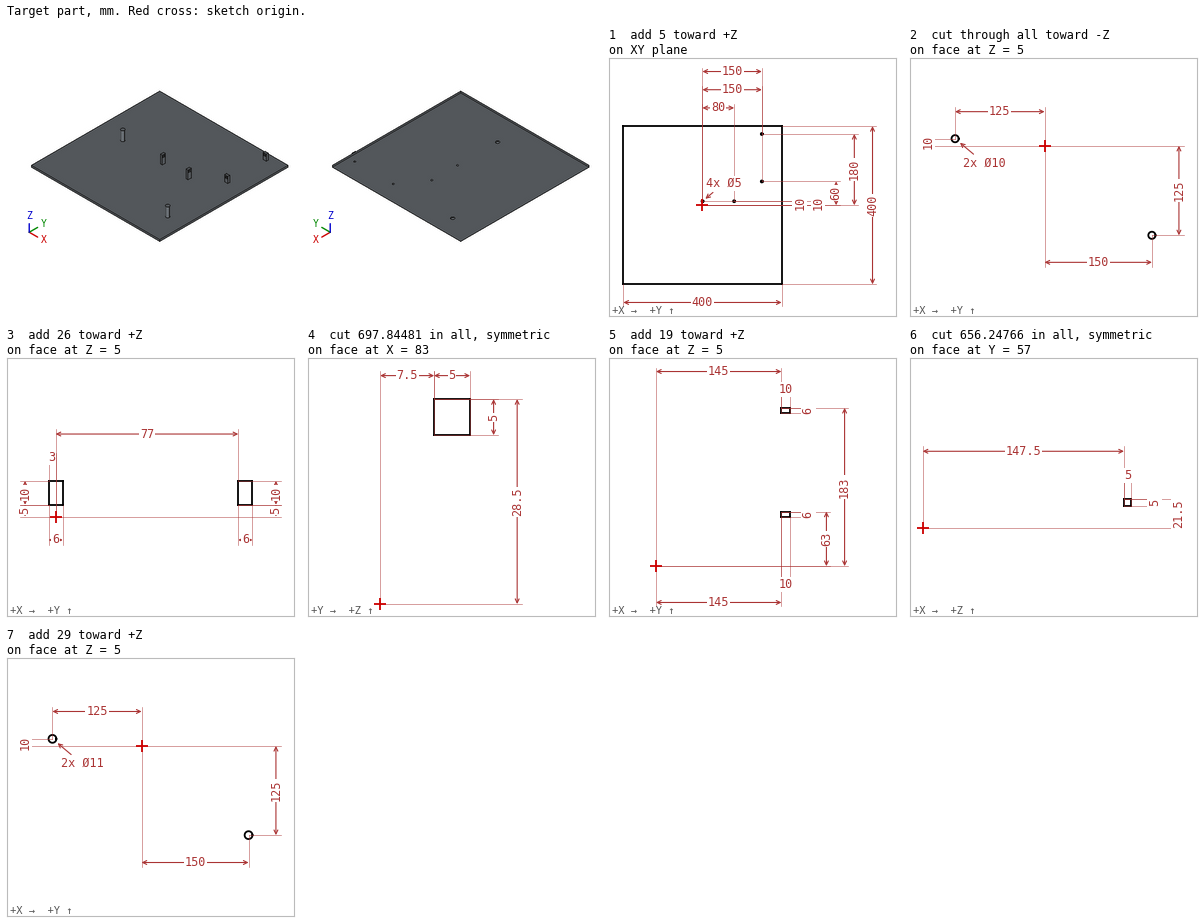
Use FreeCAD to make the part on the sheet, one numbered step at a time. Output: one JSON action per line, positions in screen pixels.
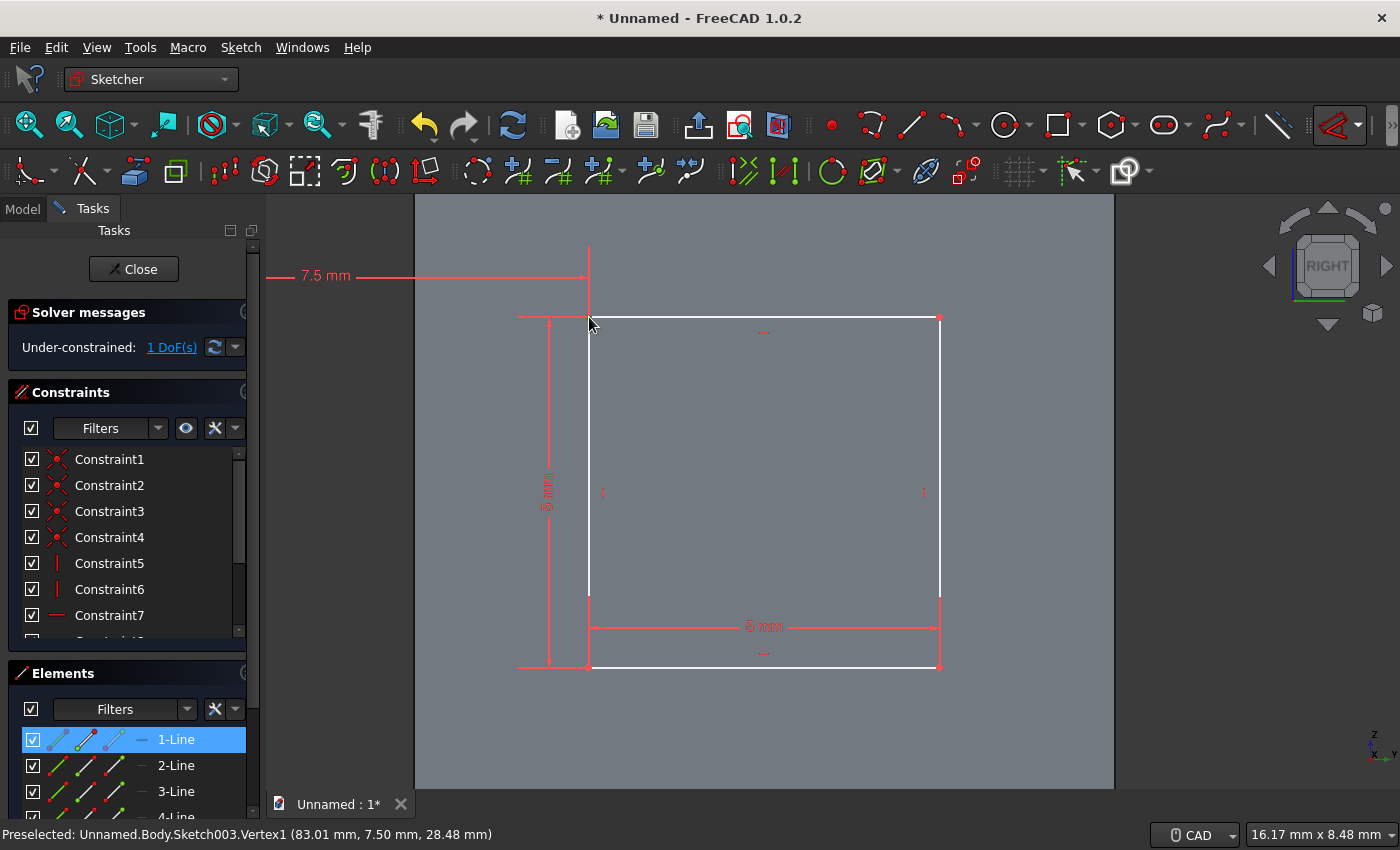
{"action": "key", "text": "i"}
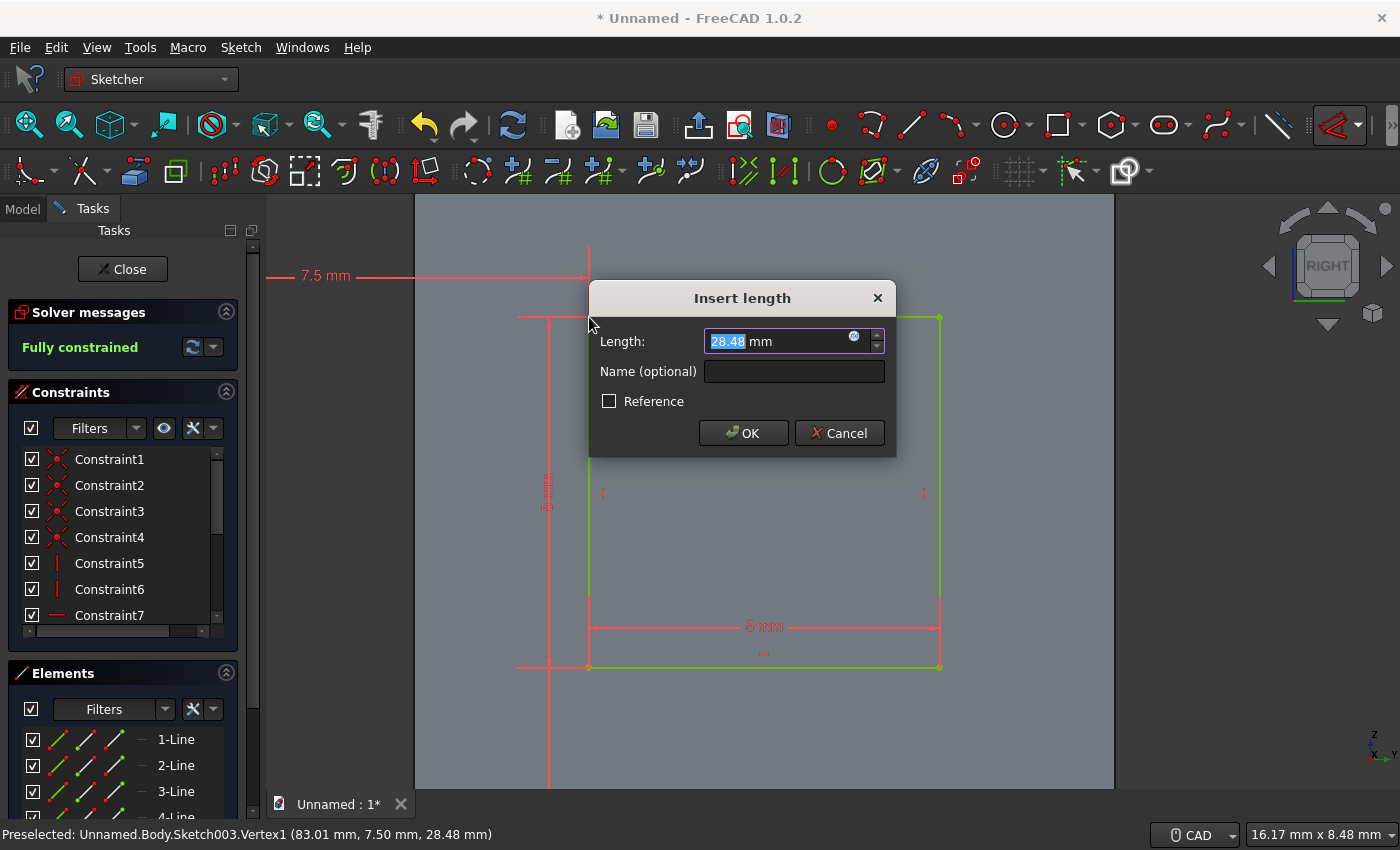
{"action": "type", "text": "28.5"}
{"action": "key", "text": "Return"}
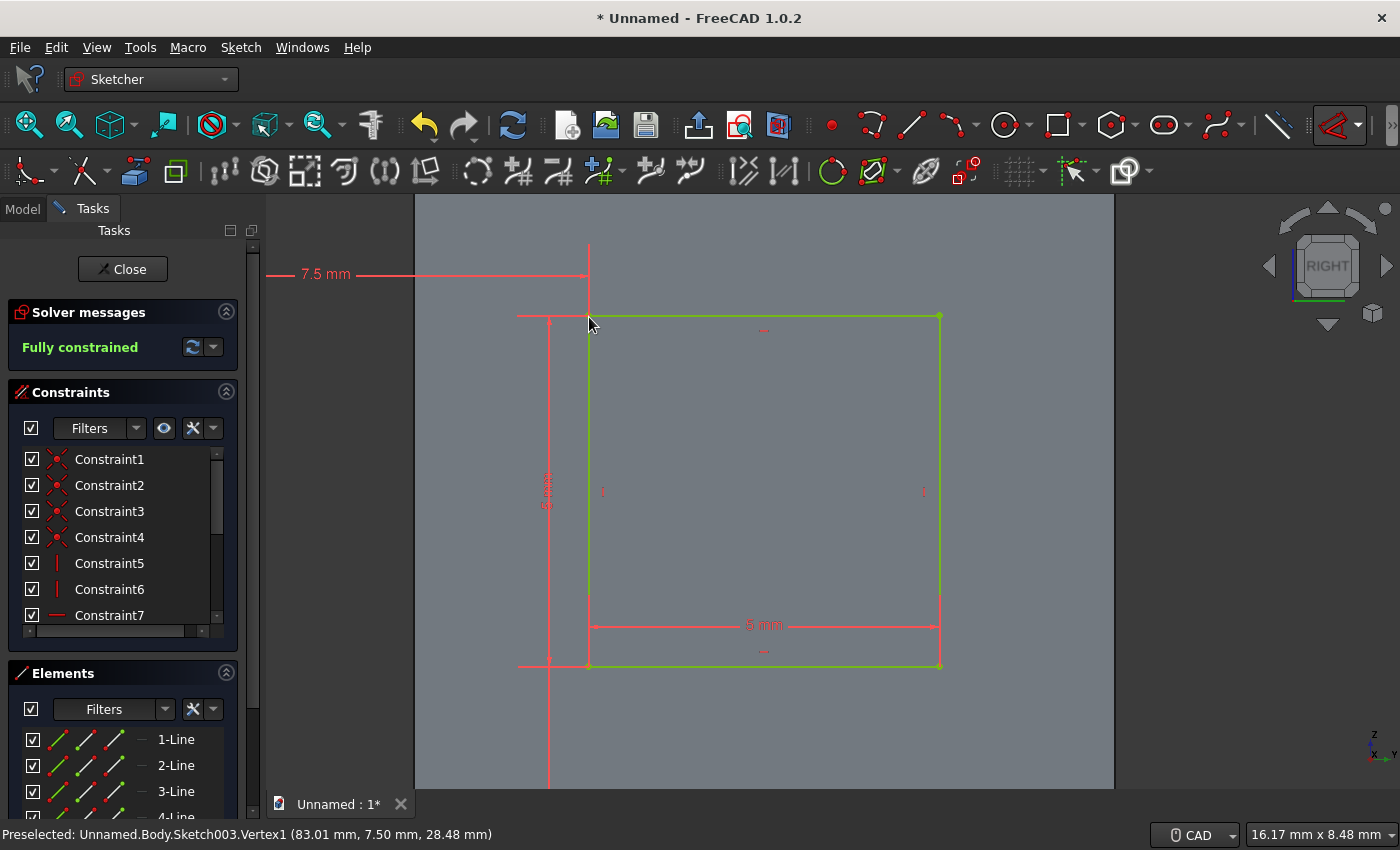
{"action": "left_click", "coordinate": [123, 269]}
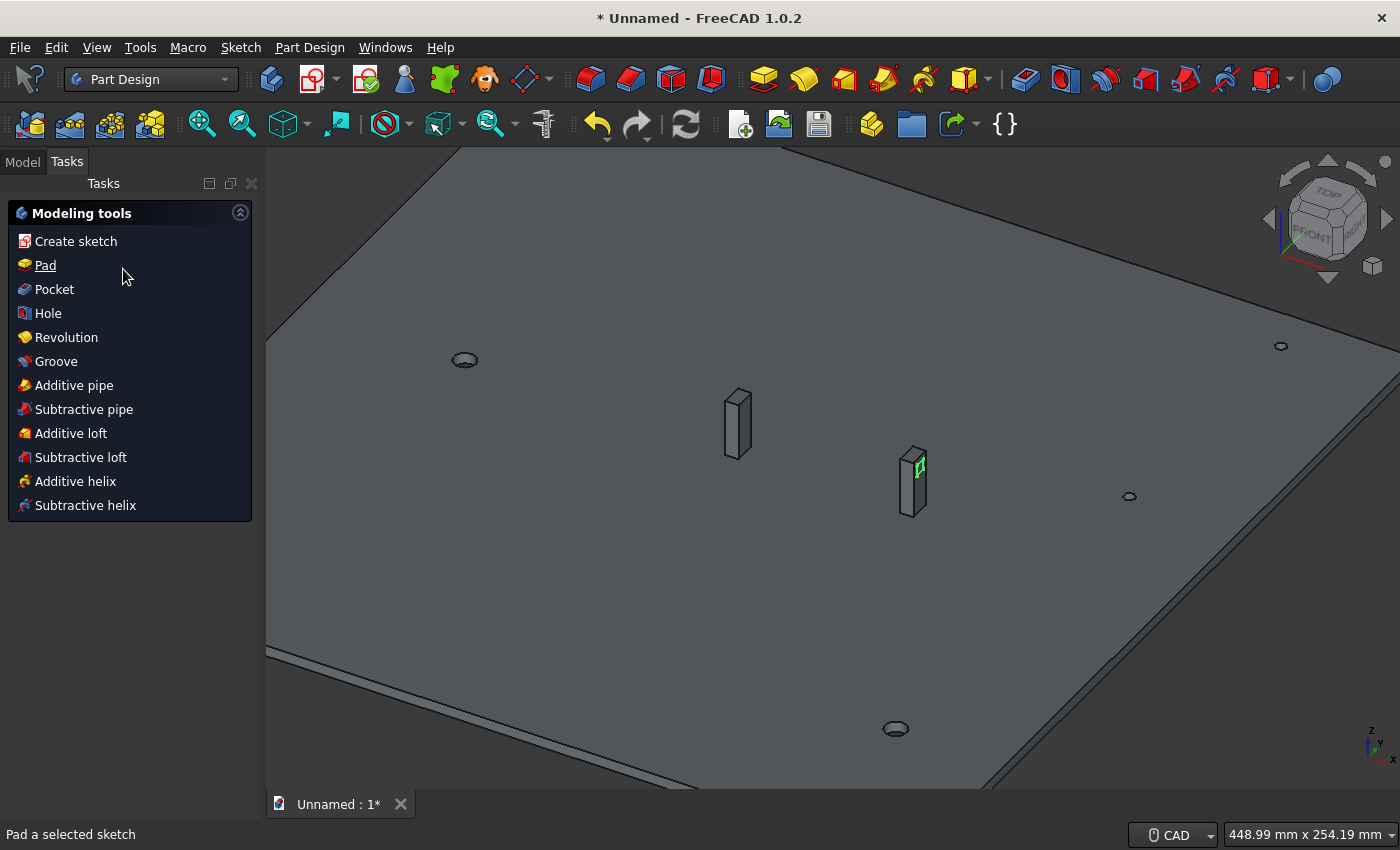
{"action": "left_click", "coordinate": [1026, 80]}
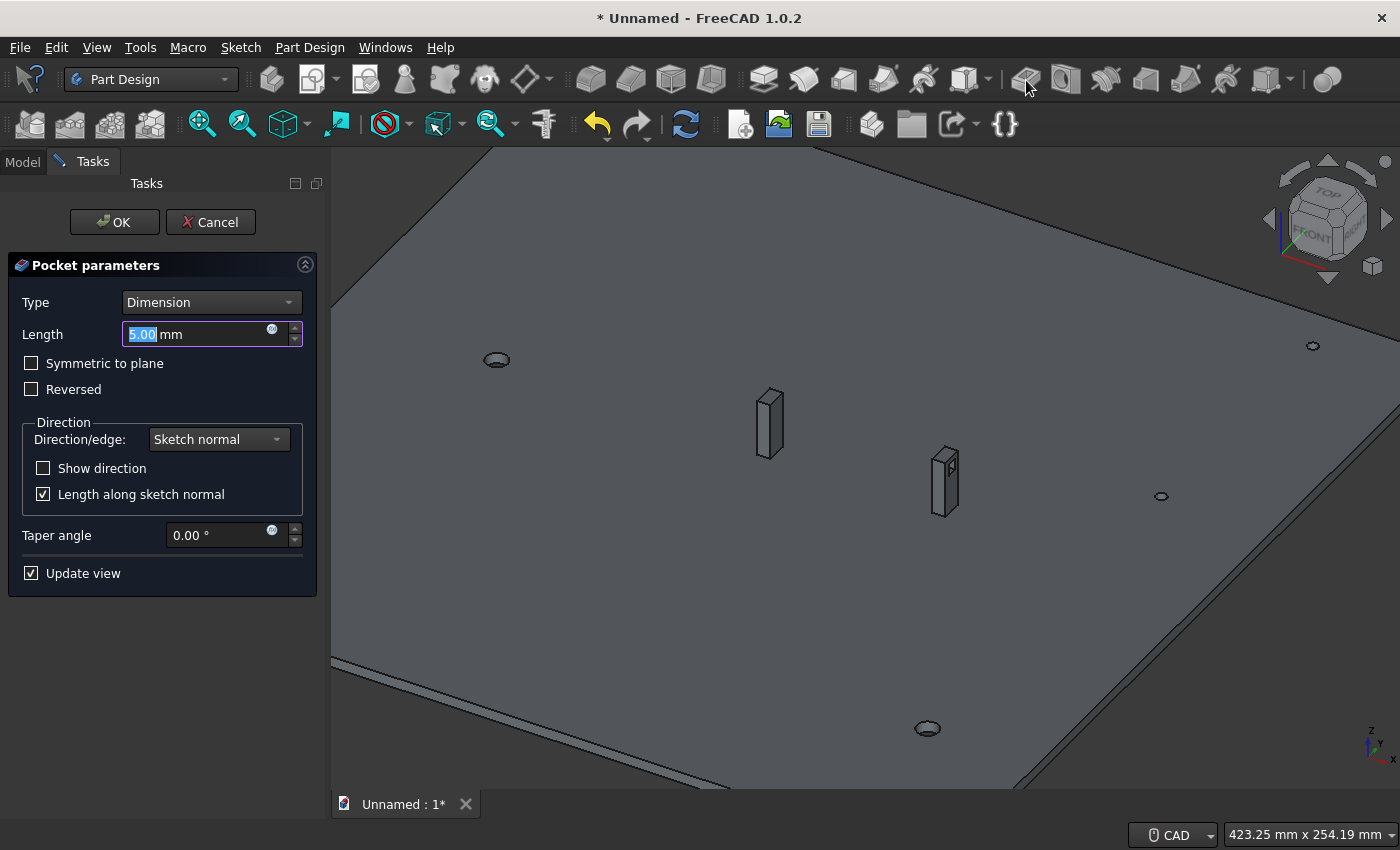
{"action": "type", "text": "697.84481"}
{"action": "key", "text": "Tab"}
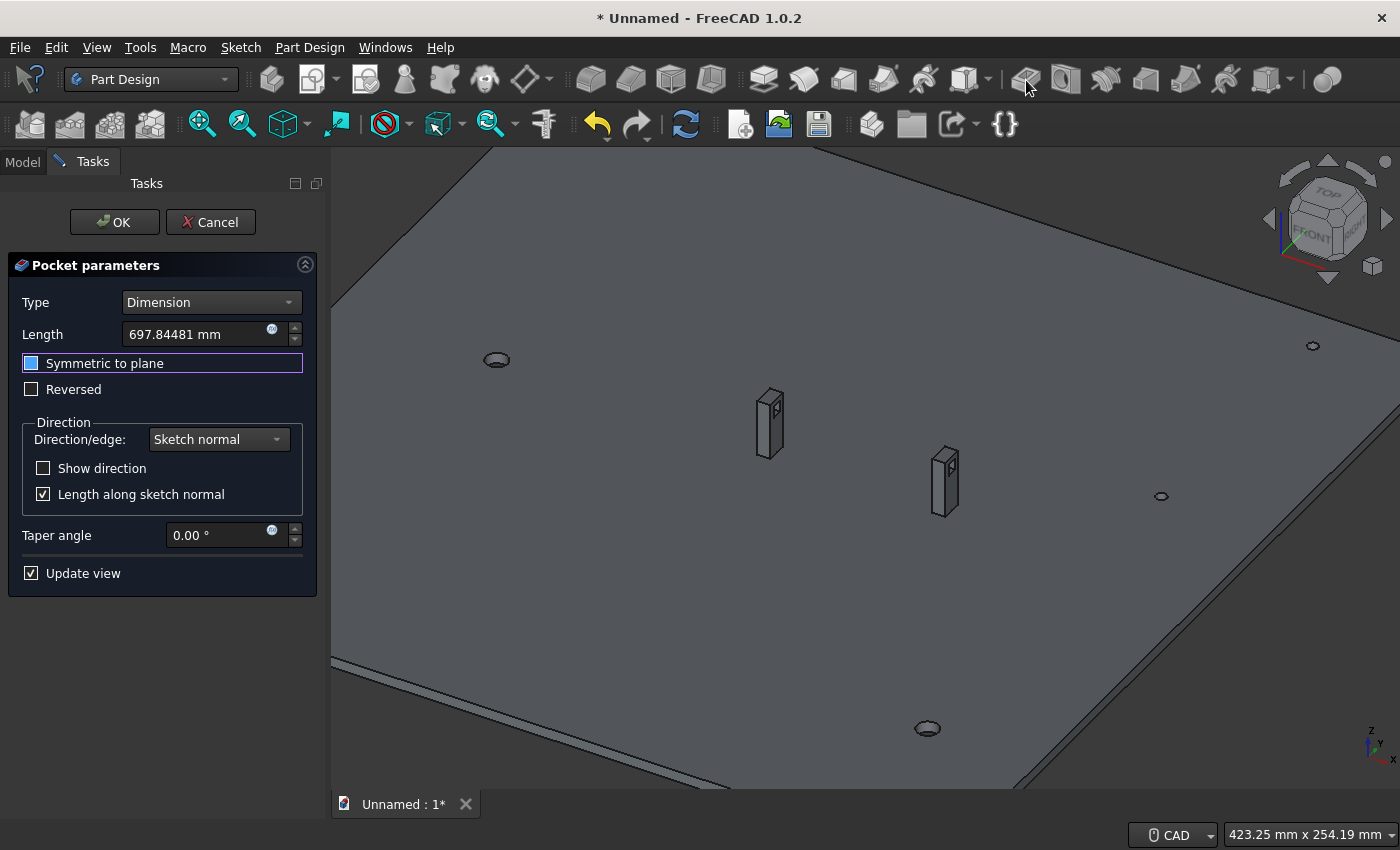
{"action": "left_click", "coordinate": [30, 363]}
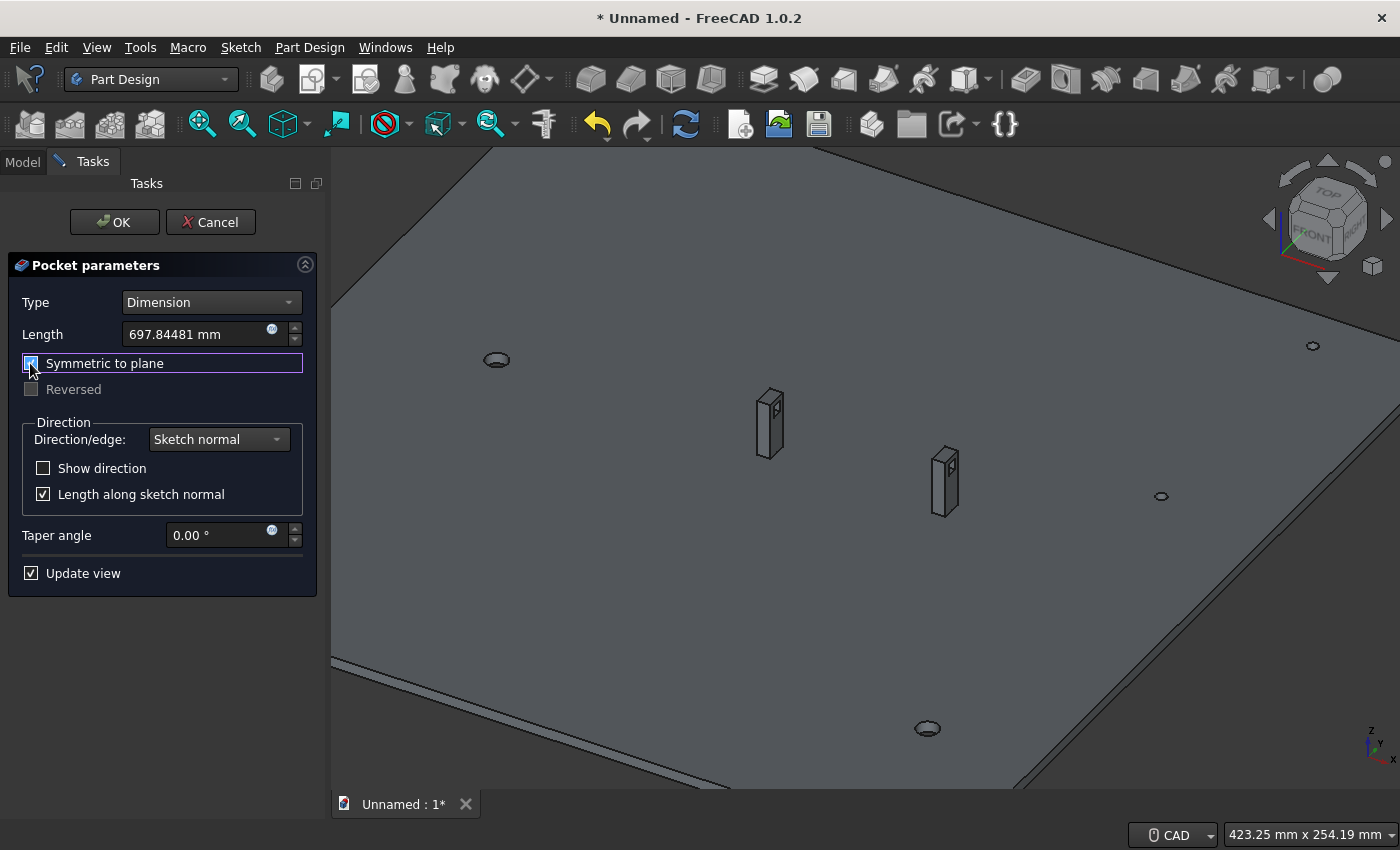
{"action": "left_click", "coordinate": [115, 222]}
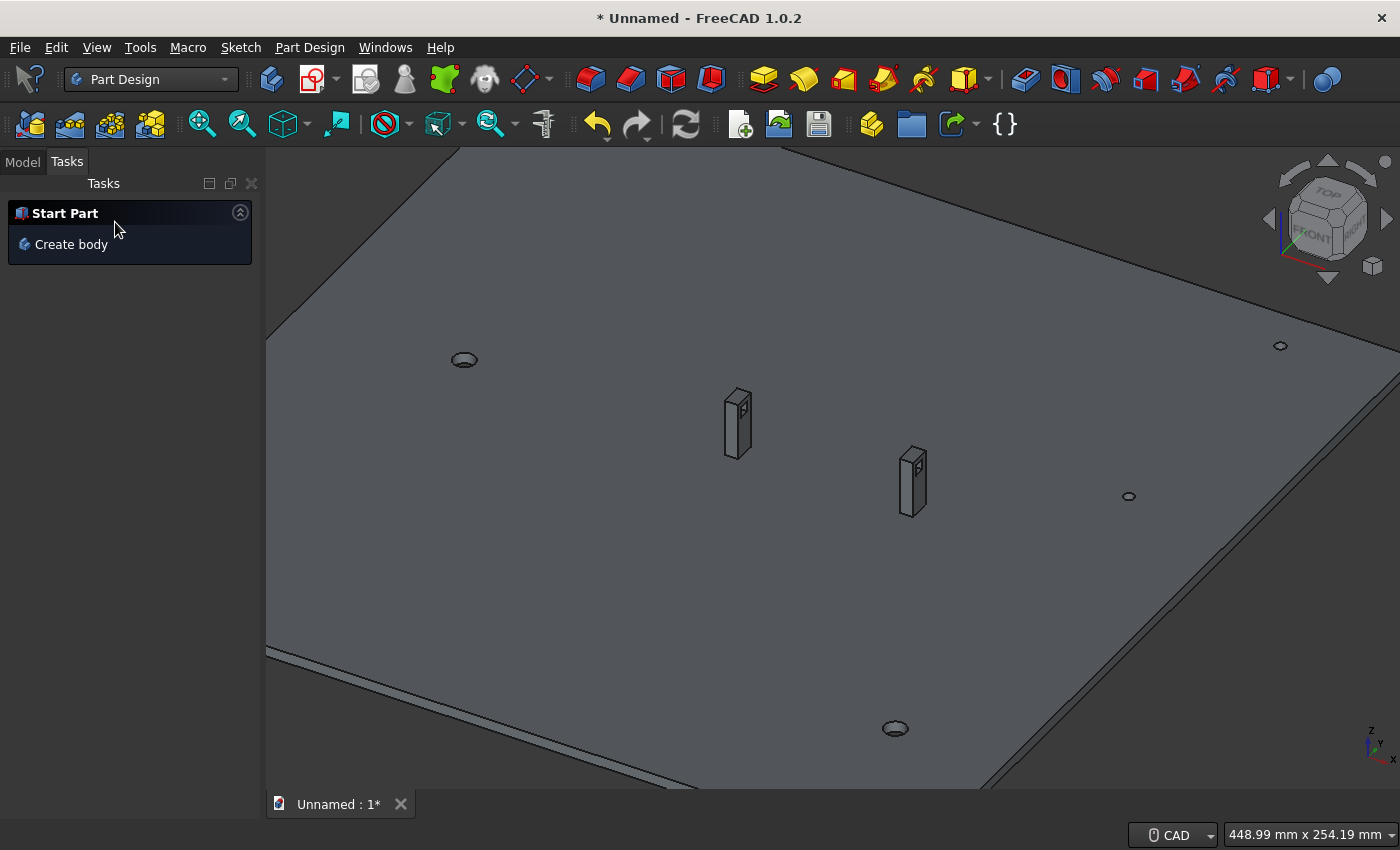
{"action": "left_click", "coordinate": [204, 124]}